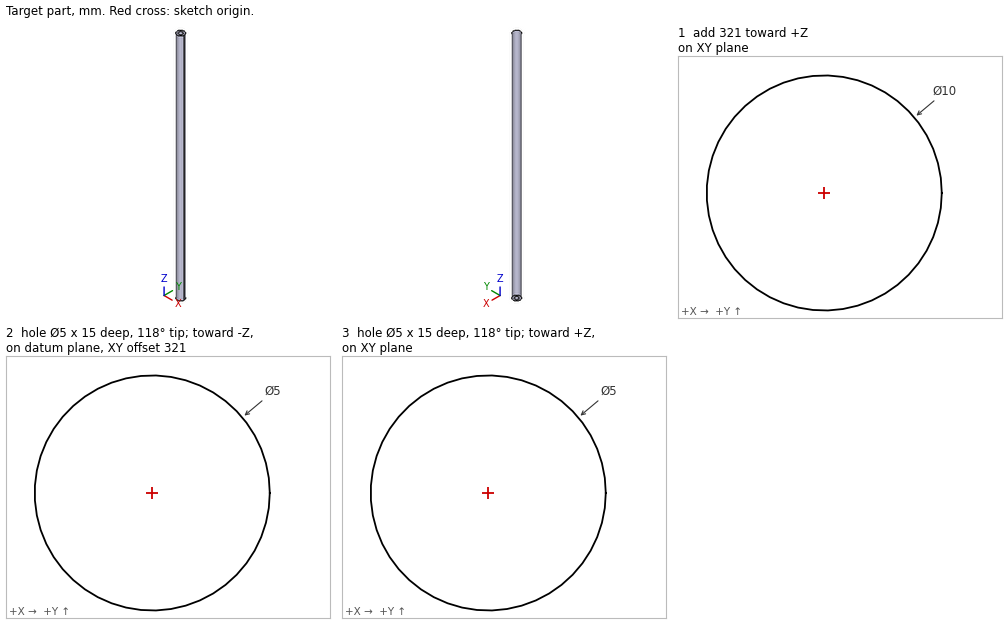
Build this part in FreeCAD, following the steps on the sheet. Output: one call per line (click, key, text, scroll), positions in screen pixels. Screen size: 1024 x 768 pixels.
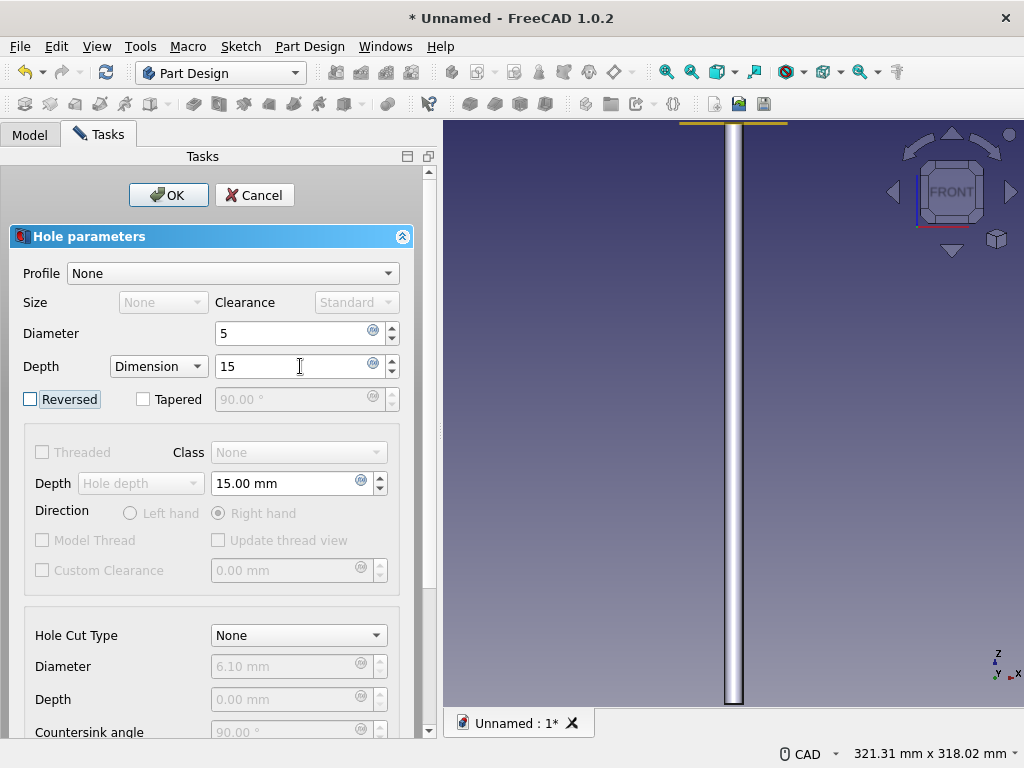
click(169, 195)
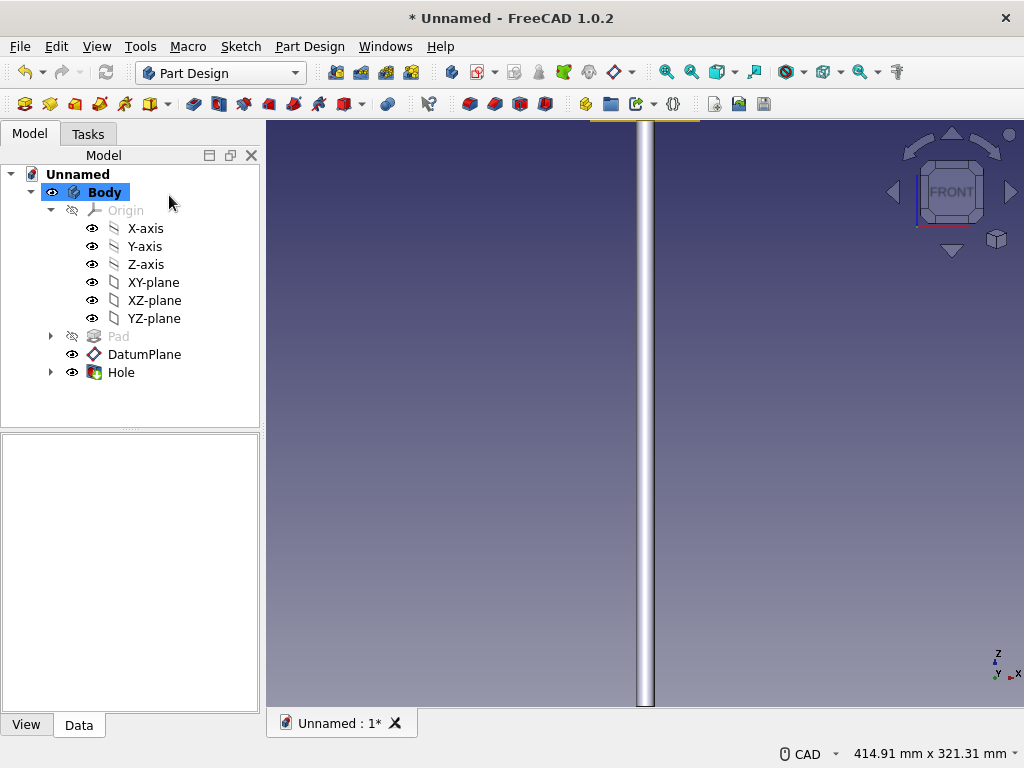
click(117, 354)
key(space)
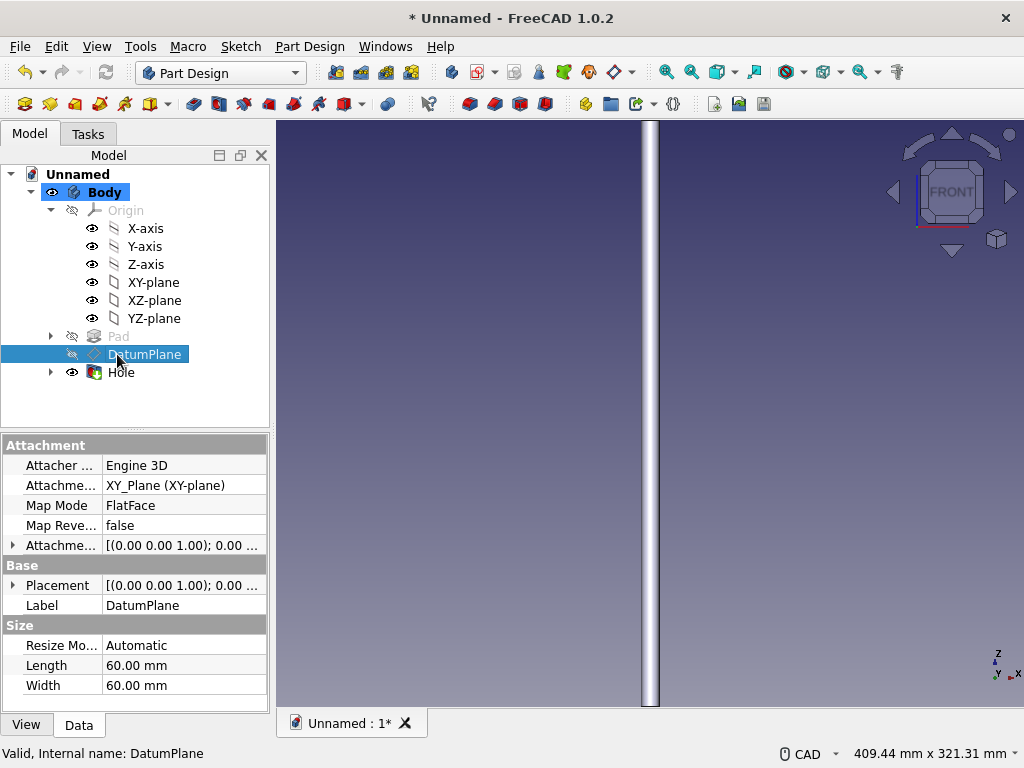
click(667, 72)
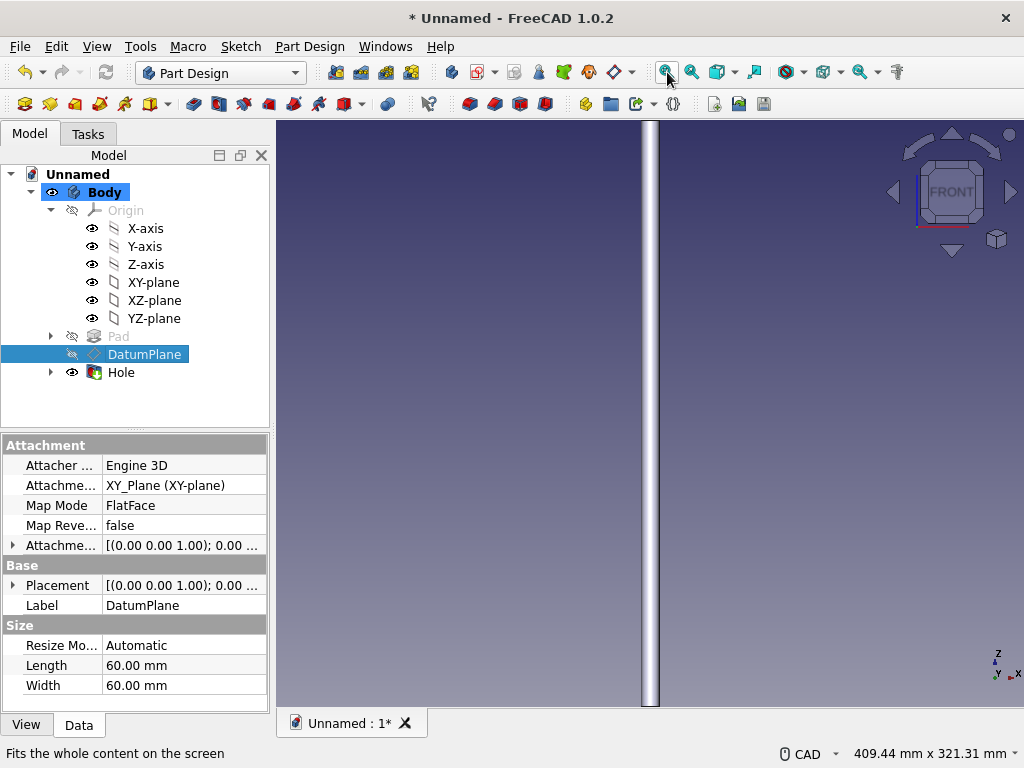
click(316, 667)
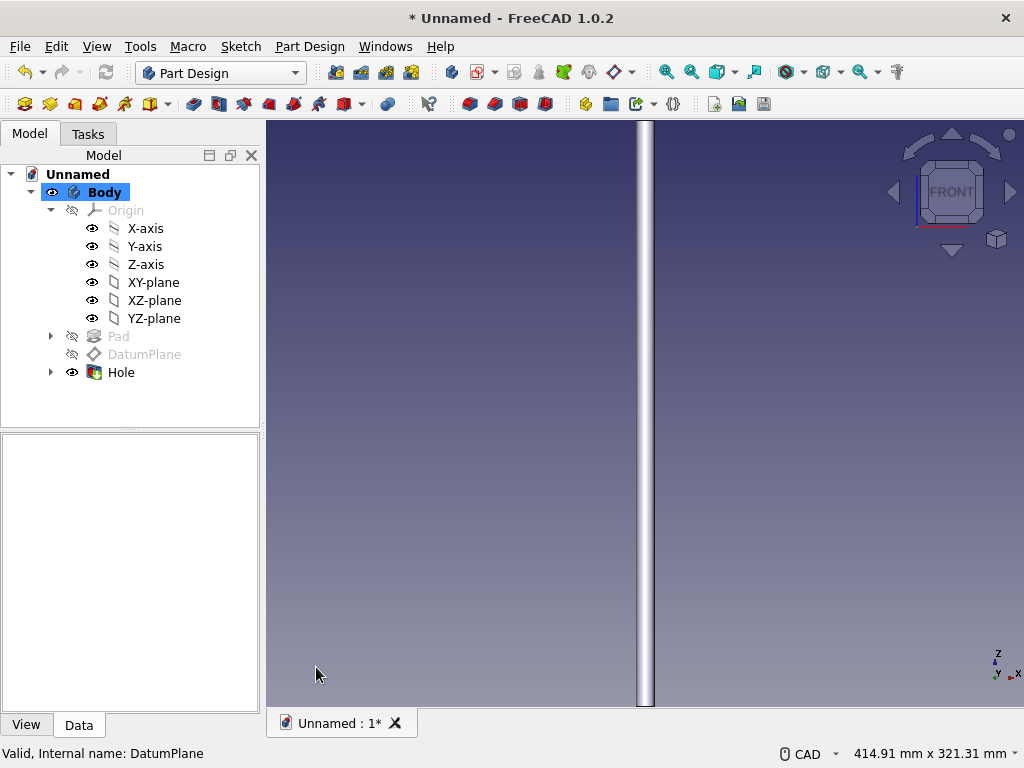
click(476, 72)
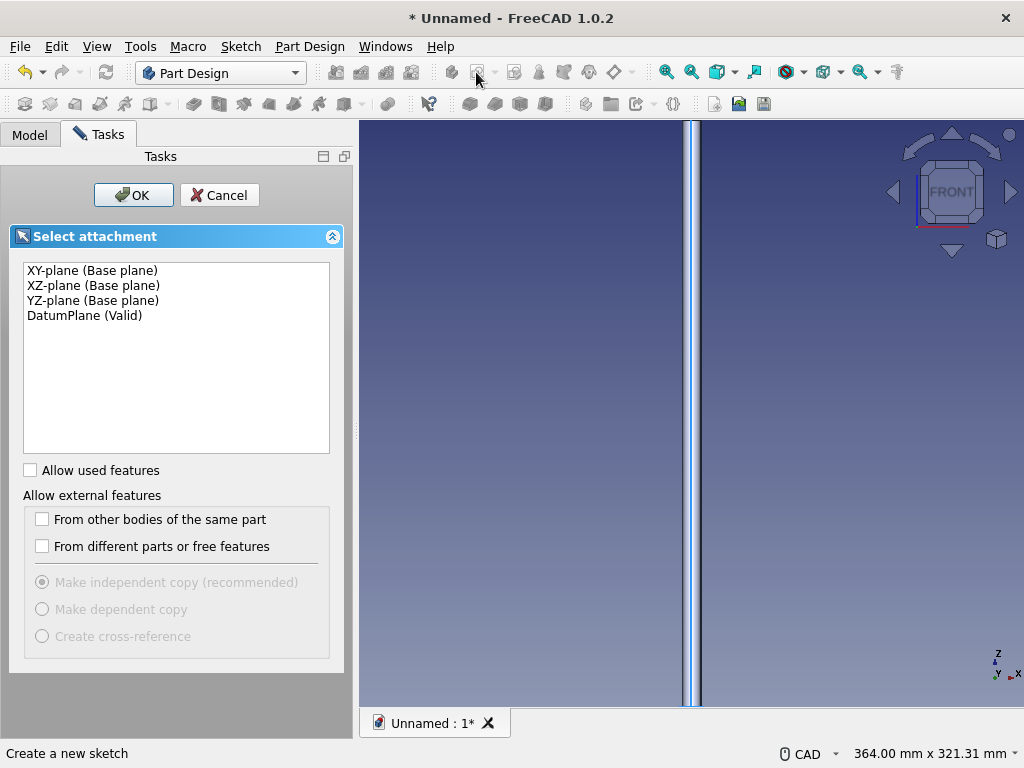
click(84, 270)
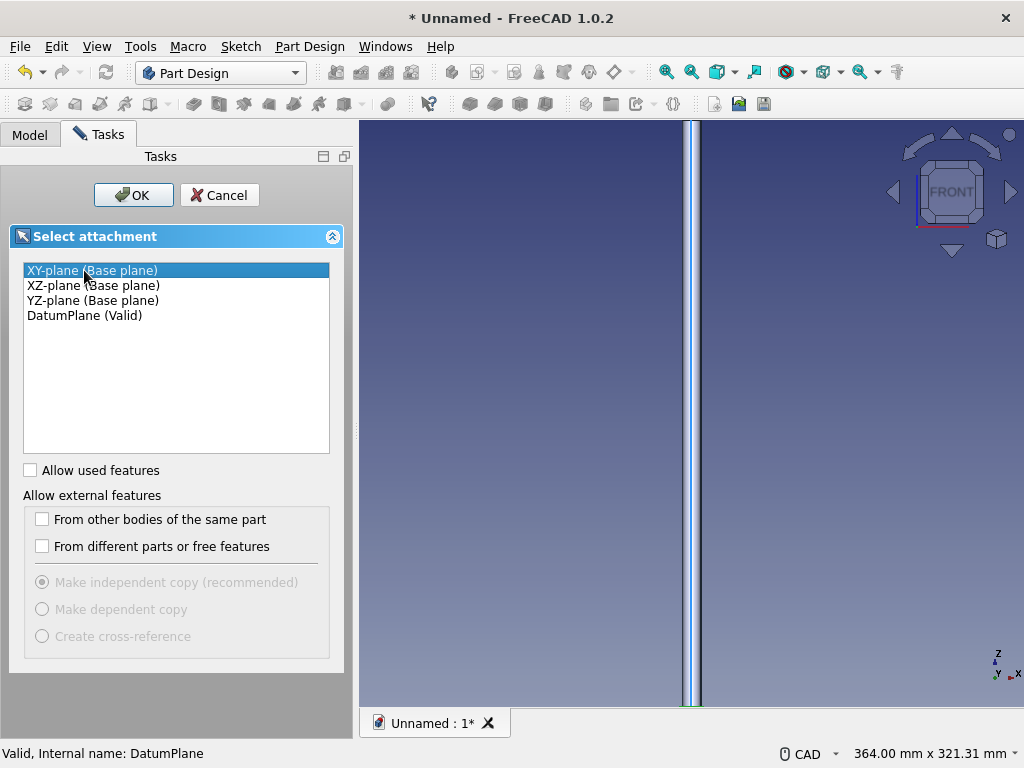
click(134, 195)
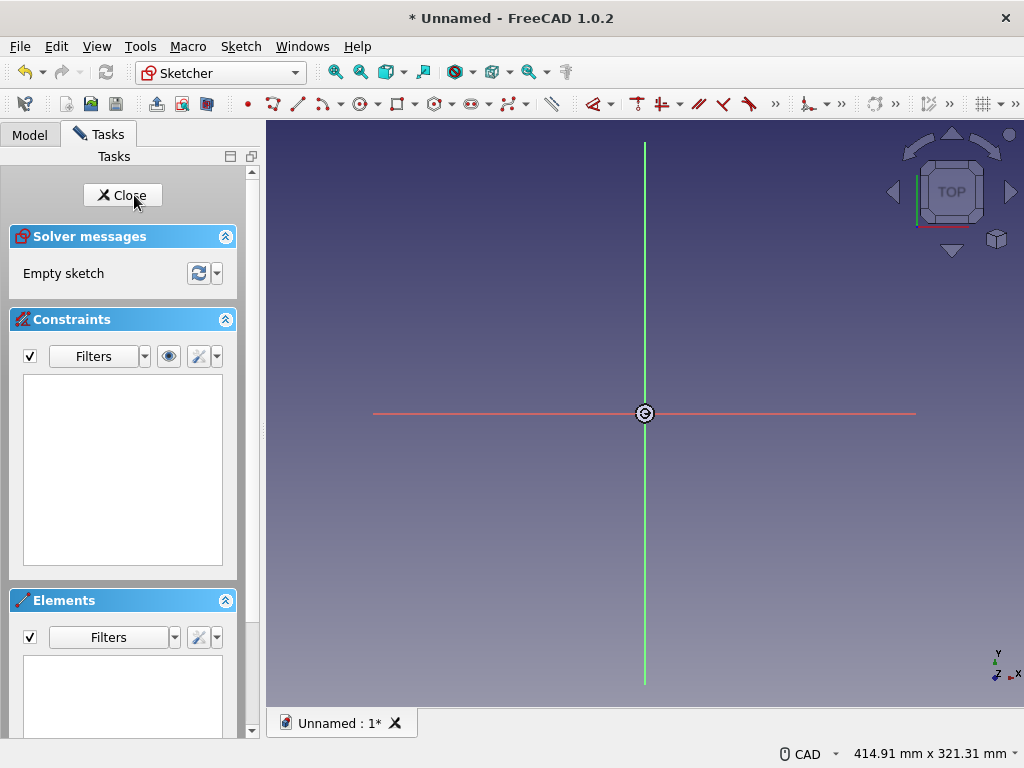
click(207, 104)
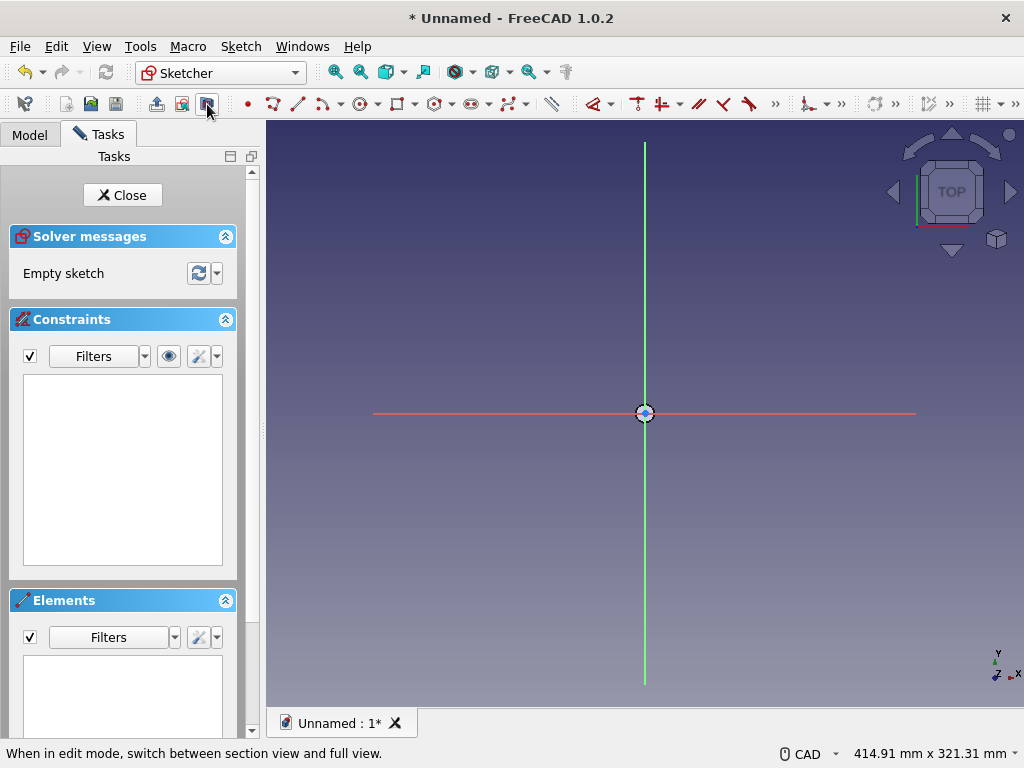
scroll(649, 414, up, 15)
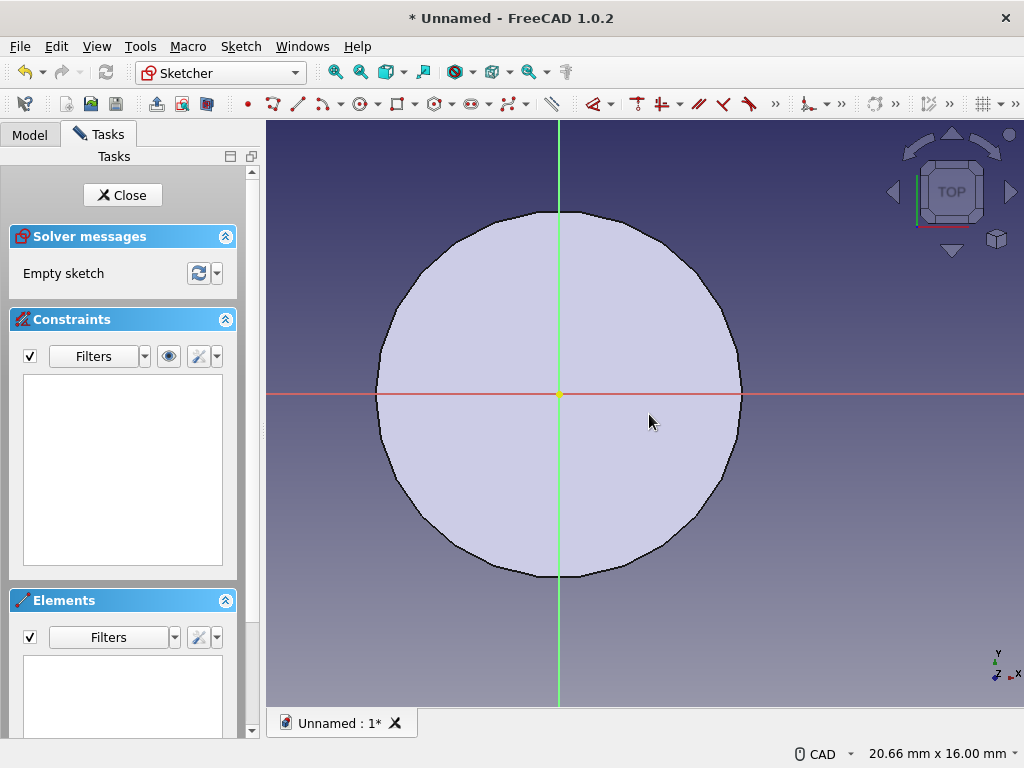
scroll(545, 379, up, 4)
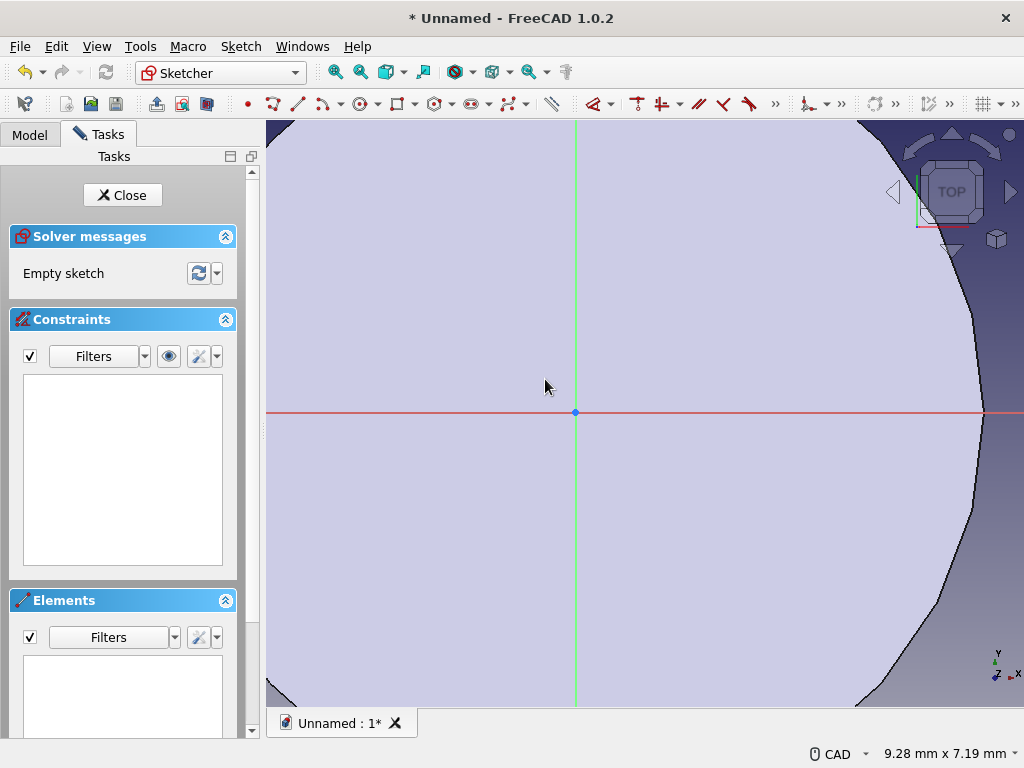
click(360, 104)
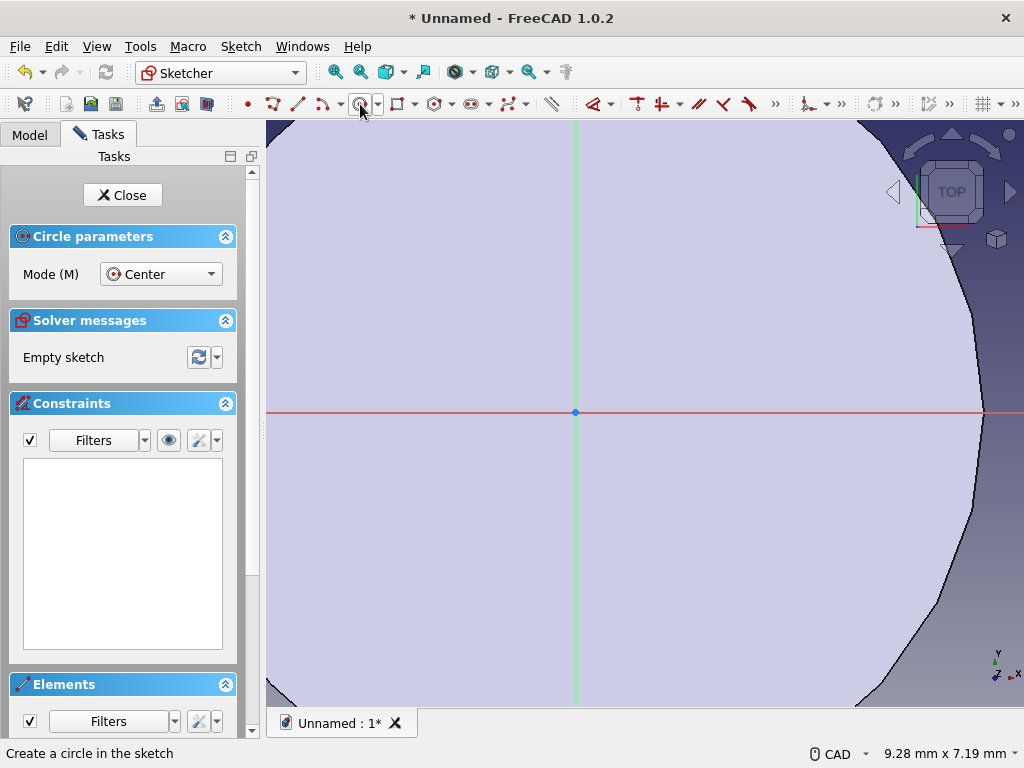
click(576, 413)
move(720, 268)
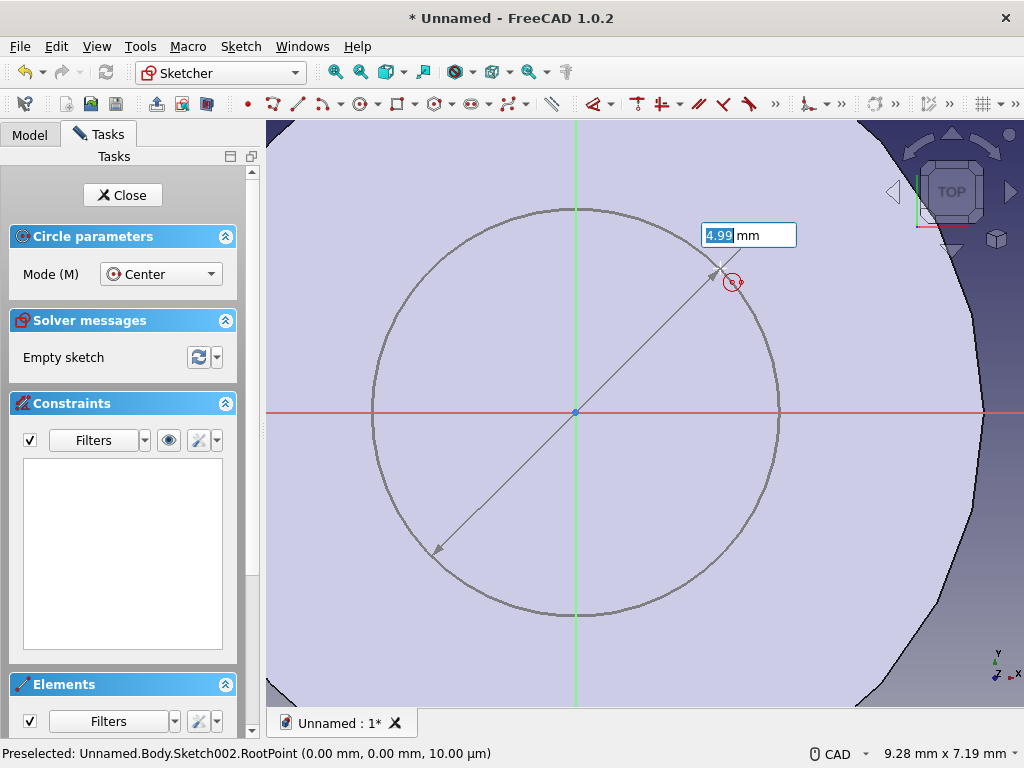
text(5)
key(Return)
key(Escape)